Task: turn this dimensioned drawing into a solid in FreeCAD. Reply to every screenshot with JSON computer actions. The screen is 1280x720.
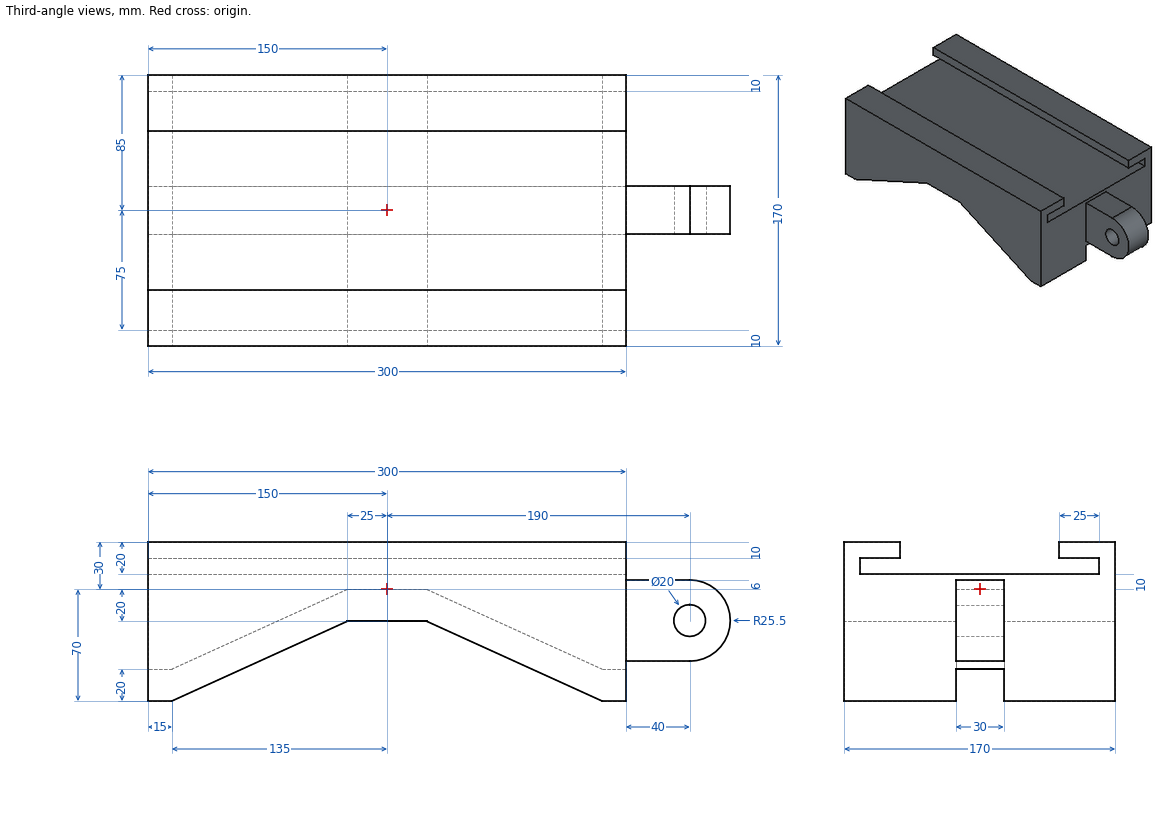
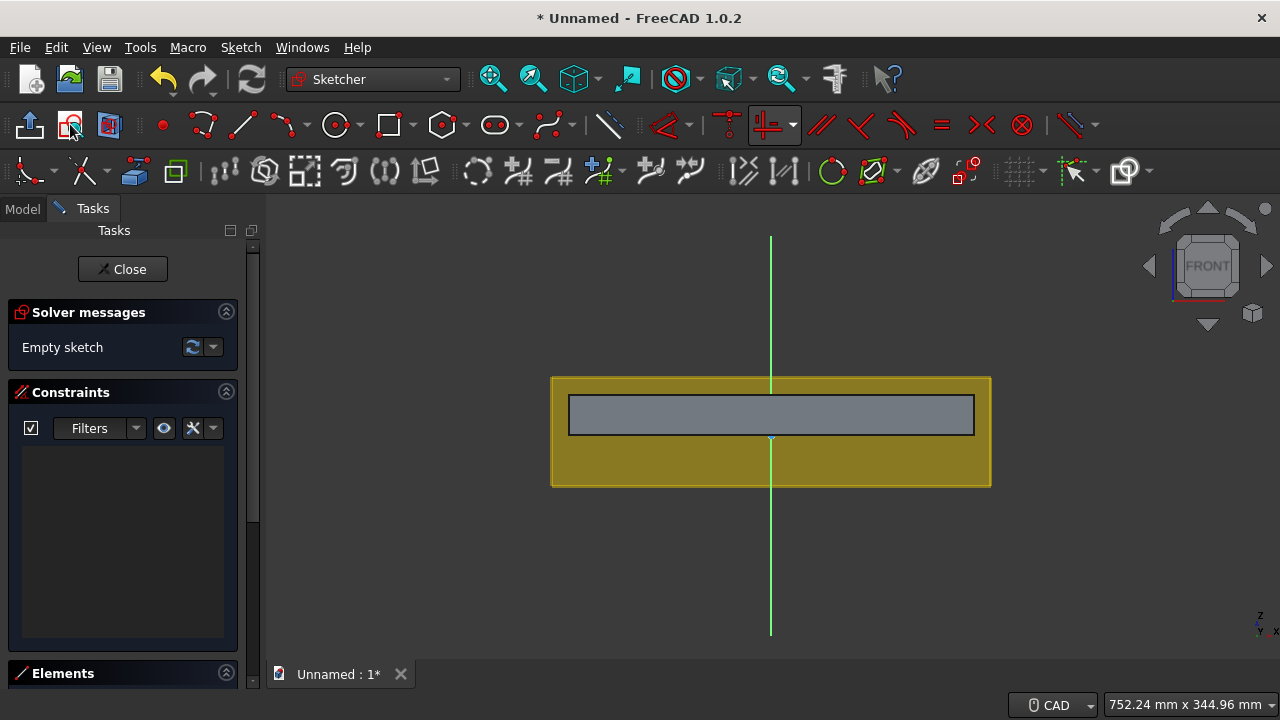
{"action": "left_click", "coordinate": [110, 126]}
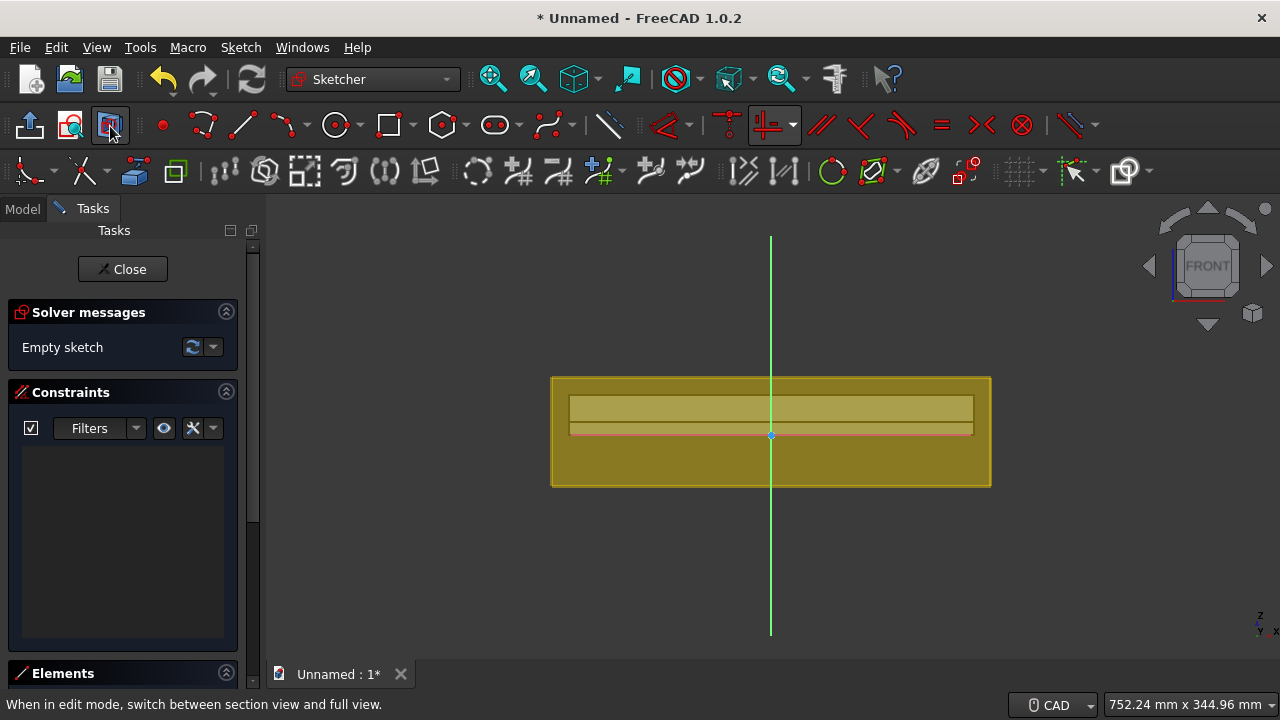
{"action": "scroll", "coordinate": [907, 392], "scroll_direction": "up", "scroll_amount": 2}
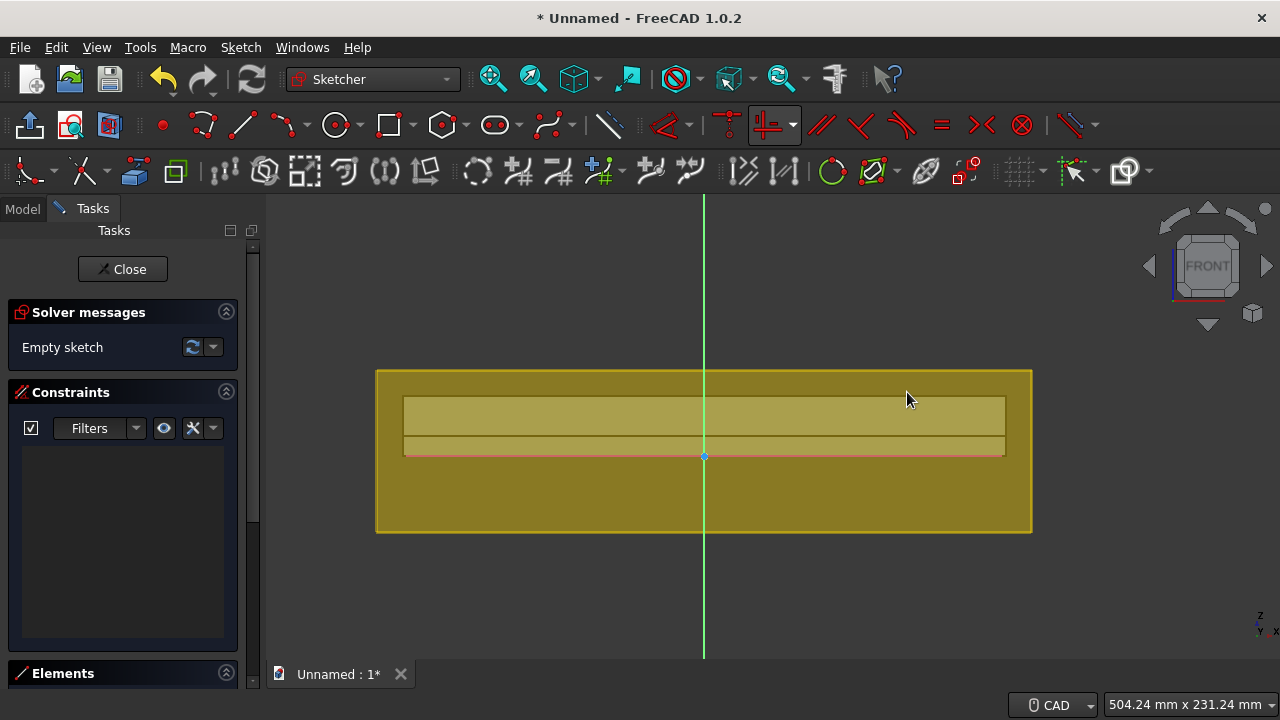
{"action": "left_click", "coordinate": [390, 126]}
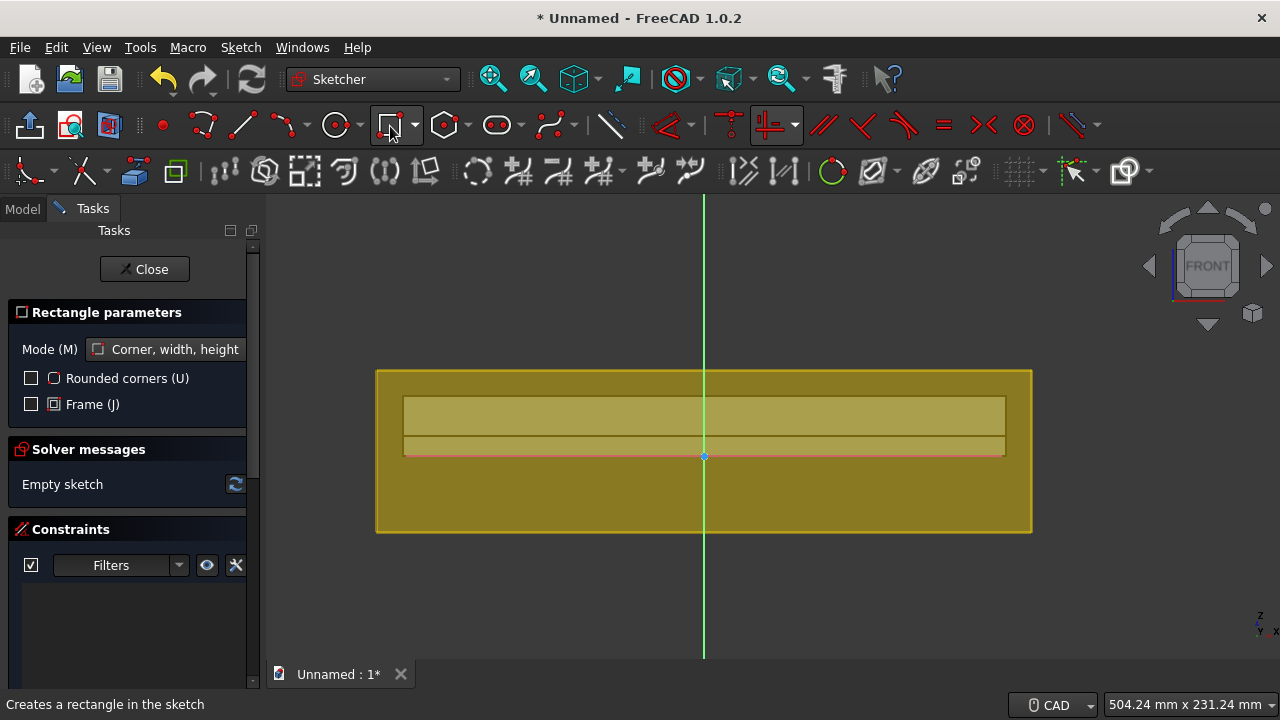
{"action": "left_click", "coordinate": [403, 396]}
{"action": "mouse_move", "coordinate": [1006, 416]}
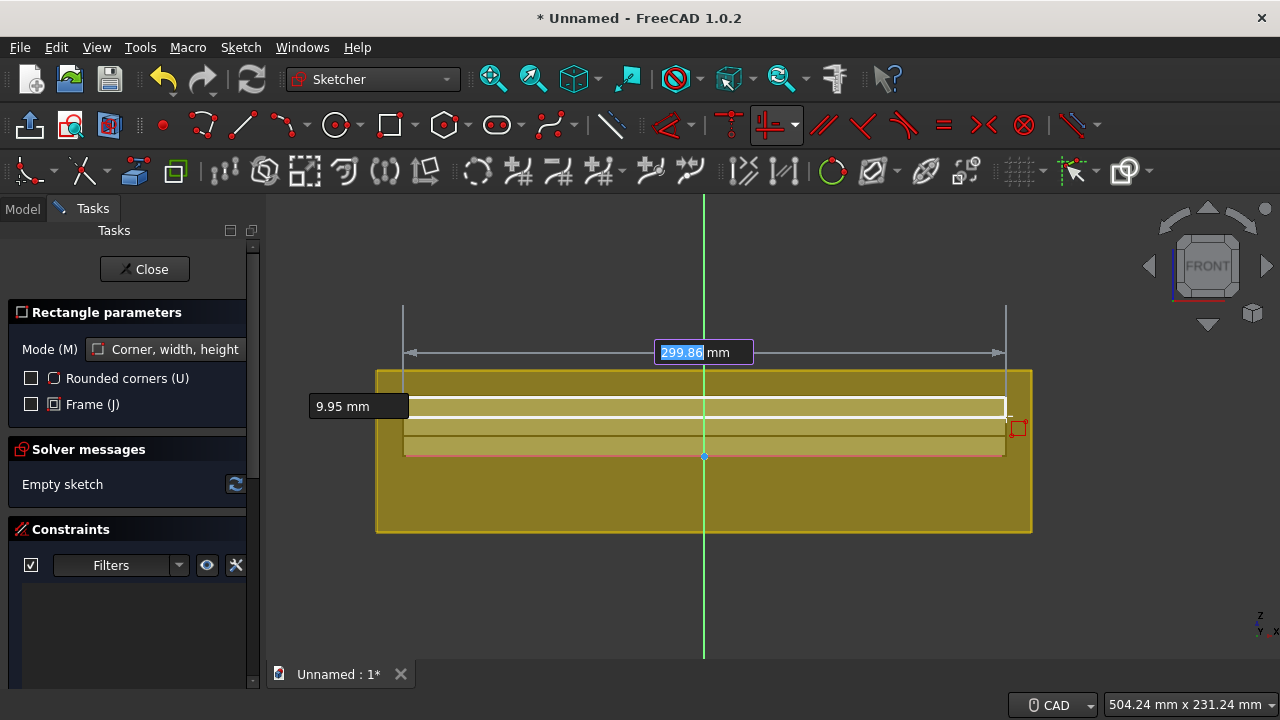
{"action": "type", "text": "300"}
{"action": "key", "text": "Tab"}
{"action": "type", "text": "10"}
{"action": "key", "text": "Return"}
{"action": "key", "text": "Escape"}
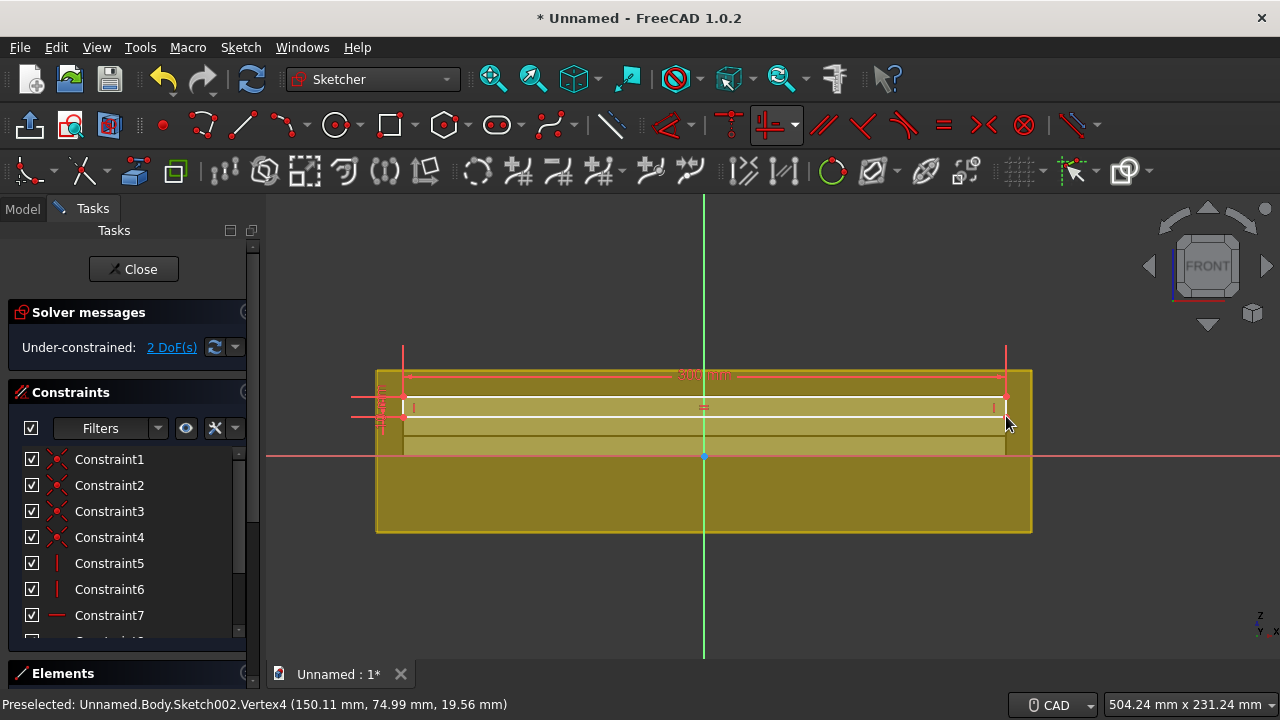
{"action": "left_click", "coordinate": [666, 126]}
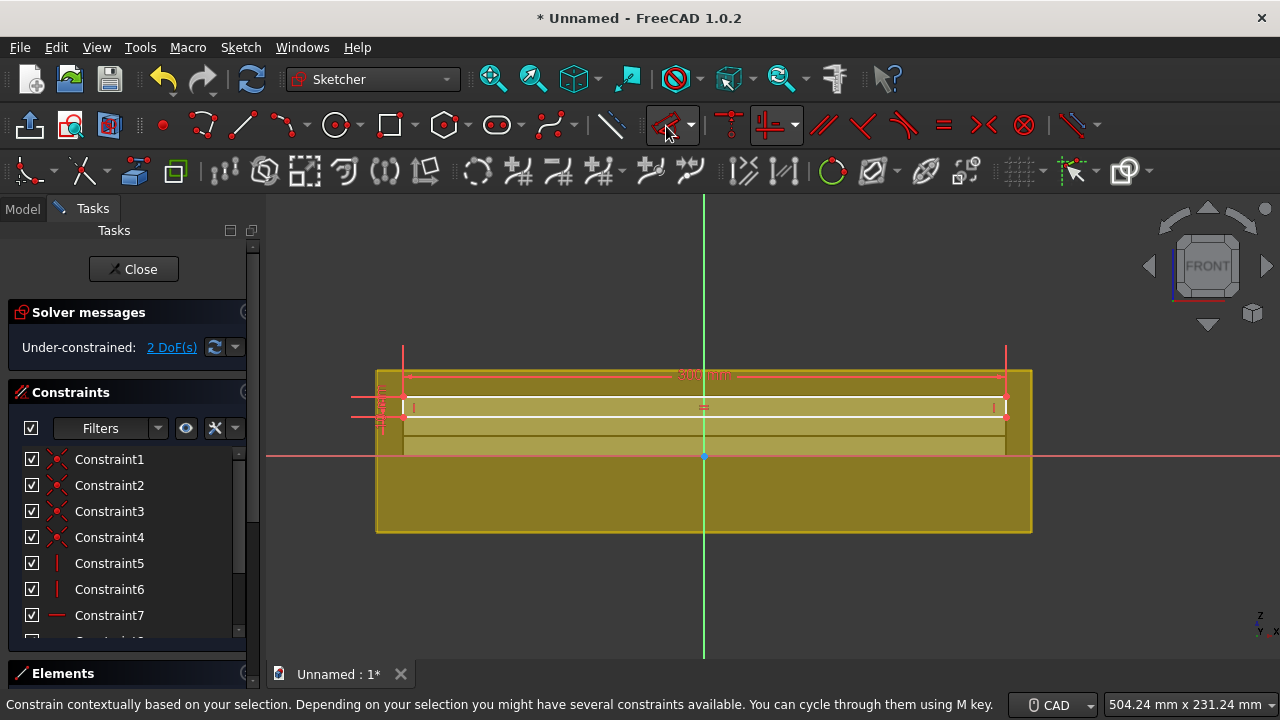
{"action": "left_click", "coordinate": [403, 397]}
{"action": "left_click", "coordinate": [369, 427]}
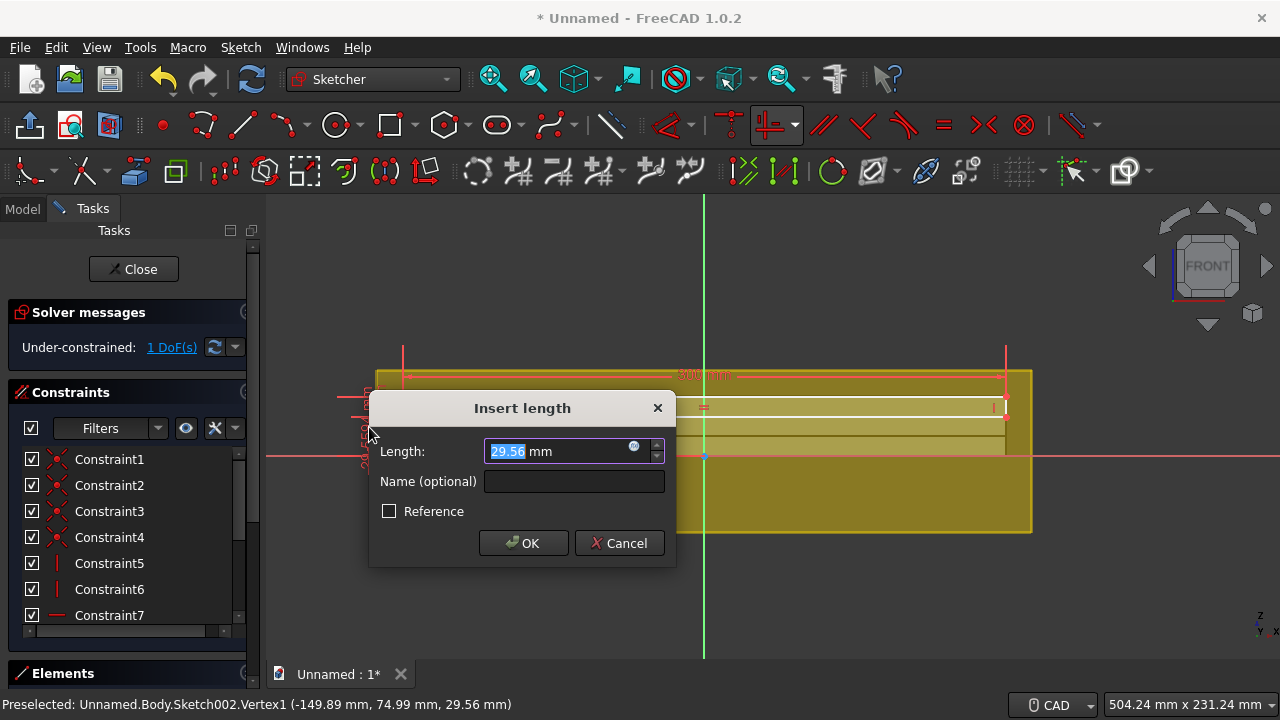
{"action": "type", "text": "30"}
{"action": "key", "text": "Return"}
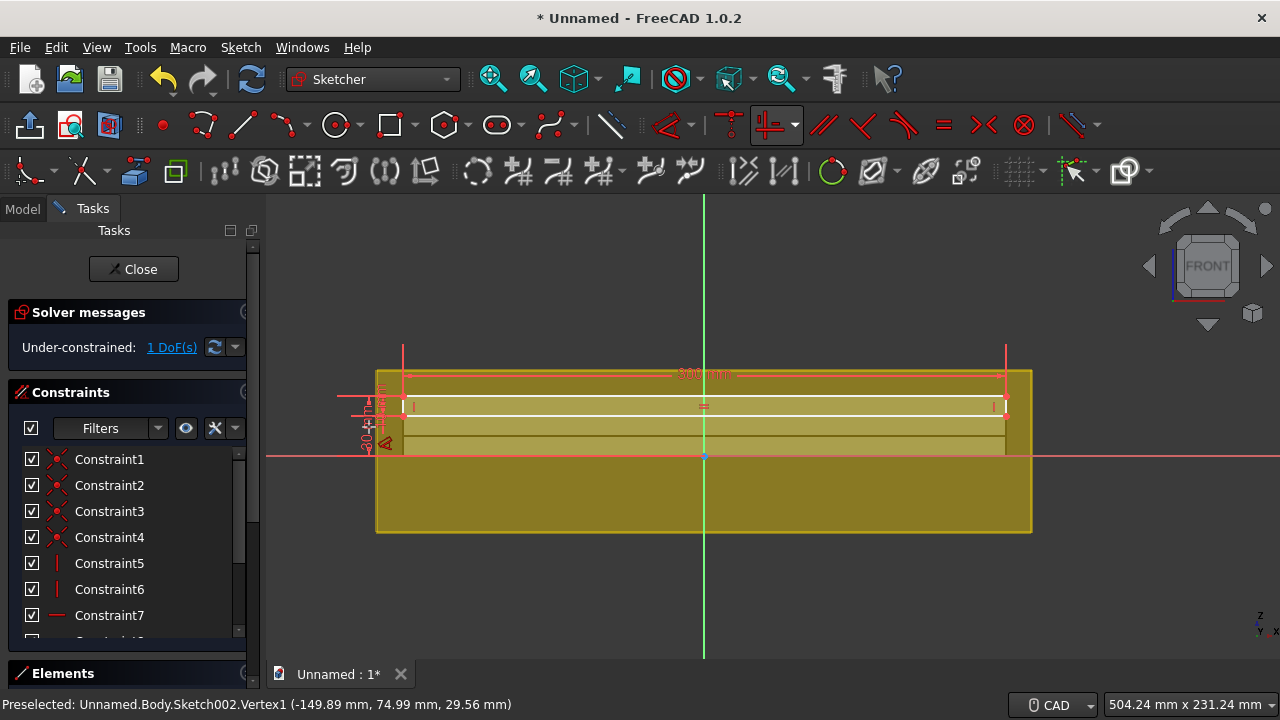
{"action": "left_click", "coordinate": [403, 396]}
{"action": "left_click", "coordinate": [554, 490]}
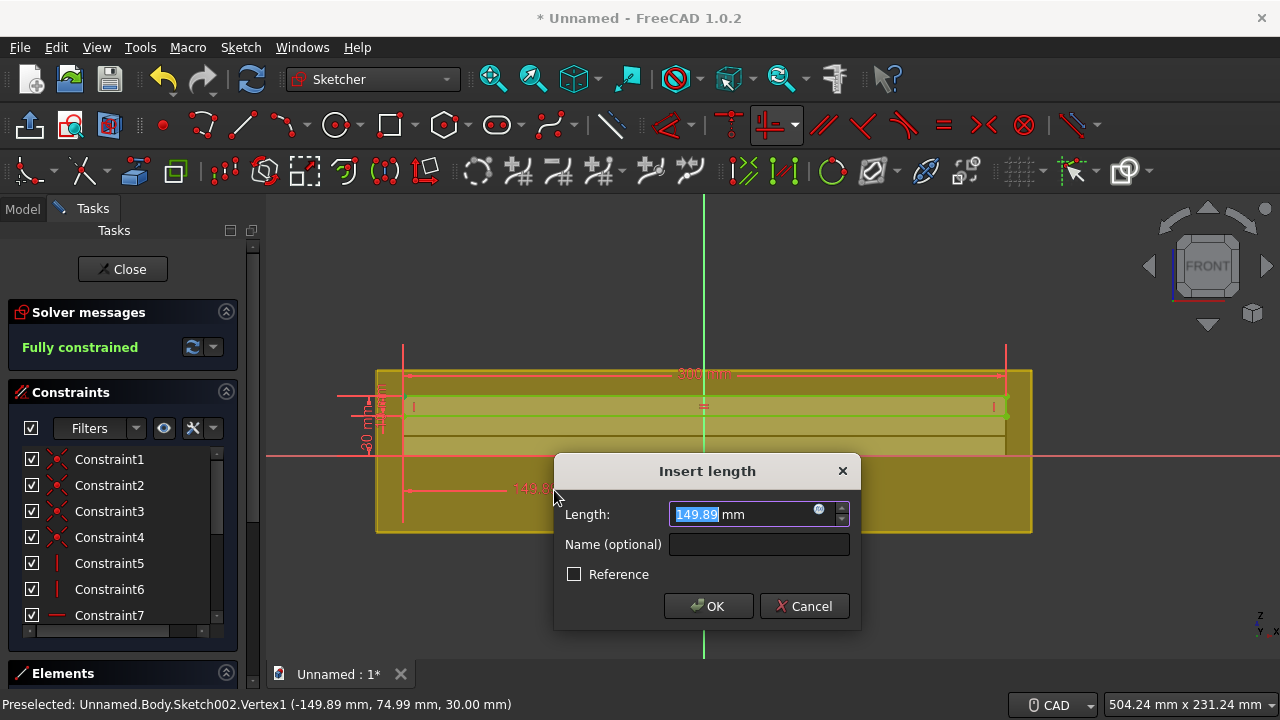
{"action": "type", "text": "150"}
{"action": "key", "text": "Return"}
{"action": "key", "text": "Escape"}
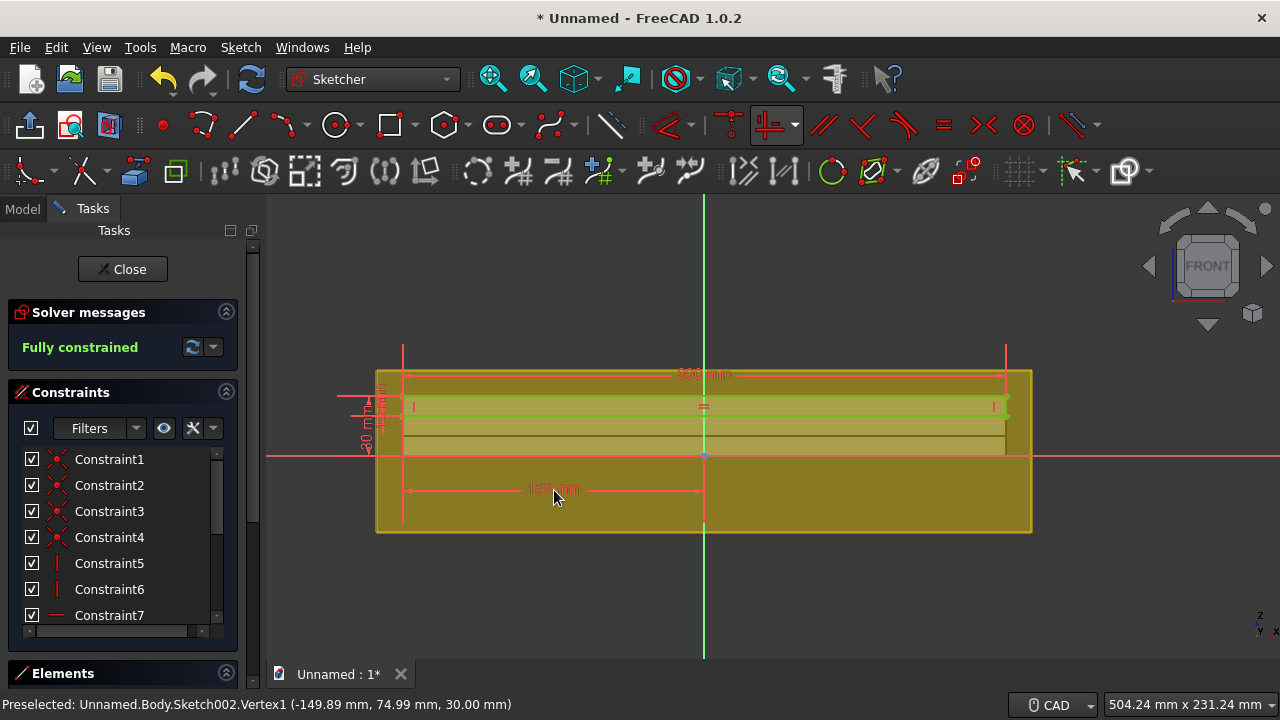
{"action": "left_click", "coordinate": [123, 269]}